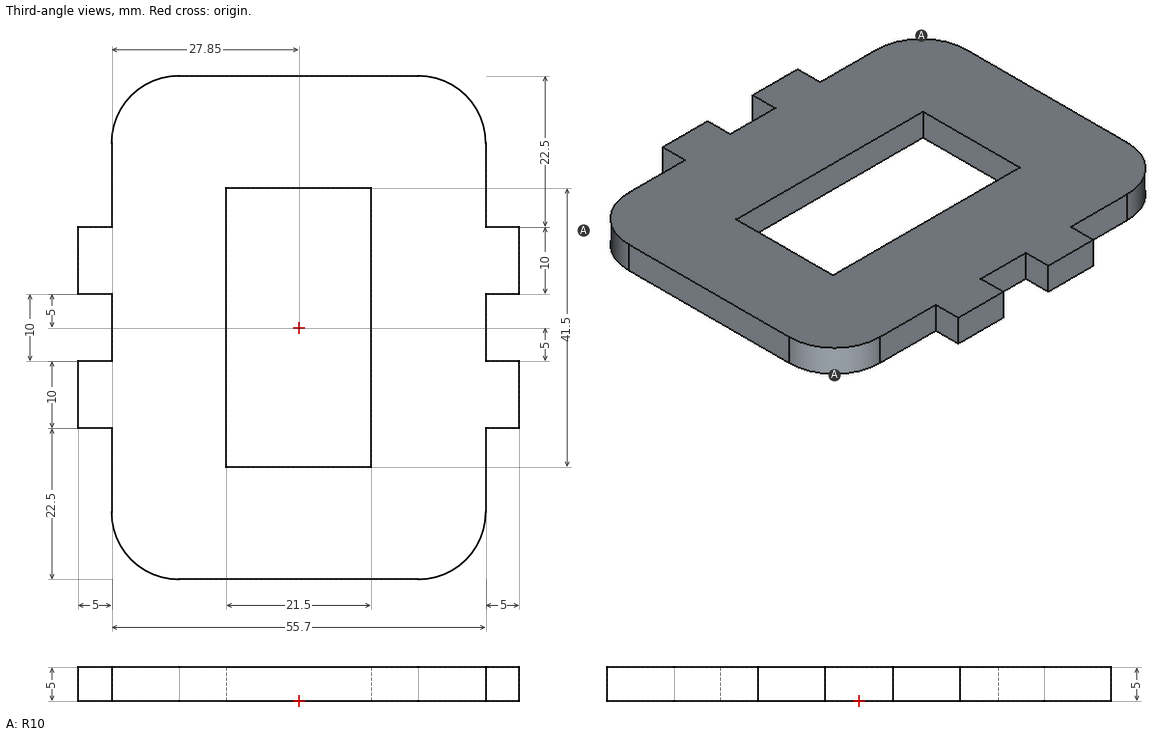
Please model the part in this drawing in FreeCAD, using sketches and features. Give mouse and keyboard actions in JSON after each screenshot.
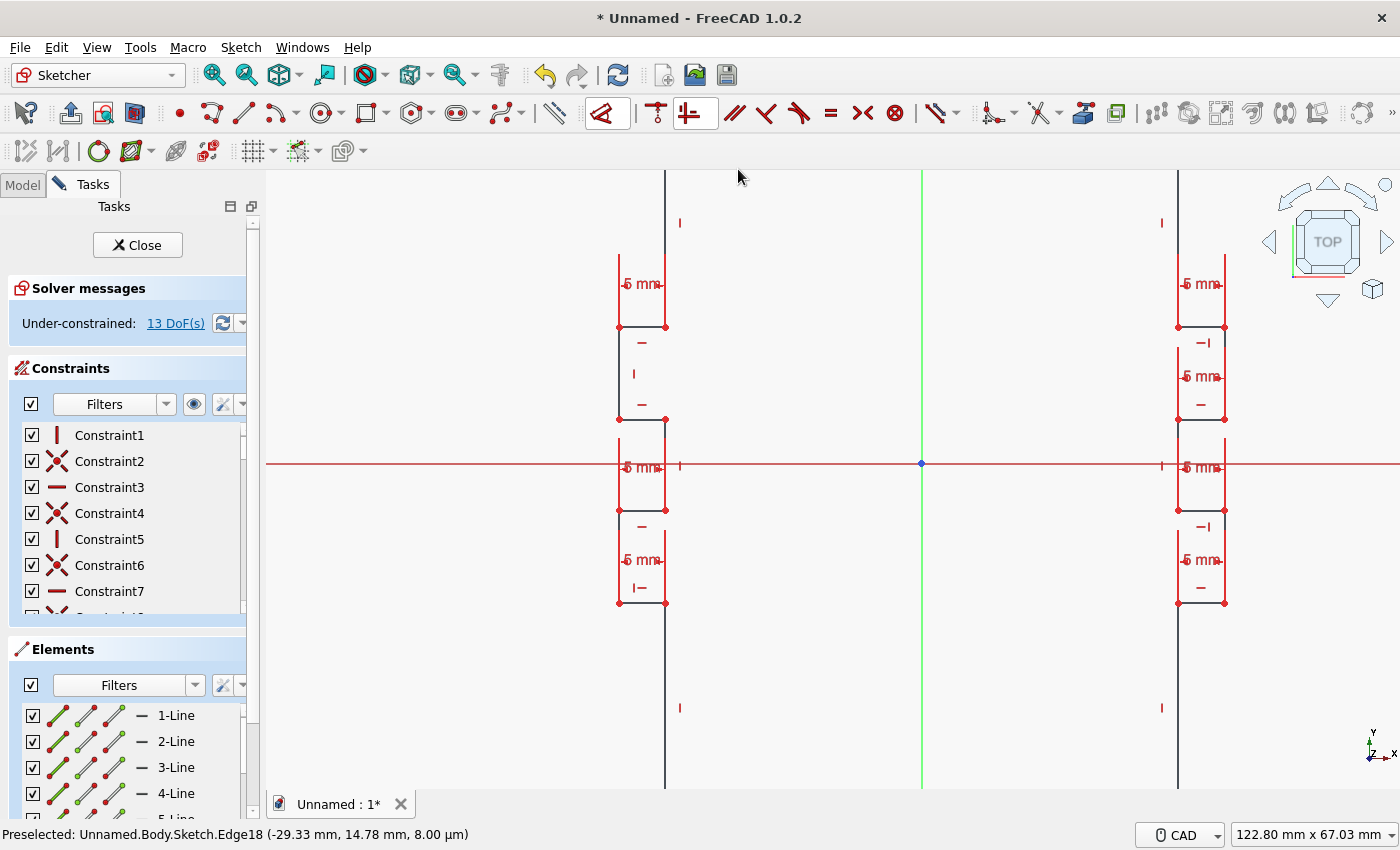
{"action": "left_click", "coordinate": [633, 420]}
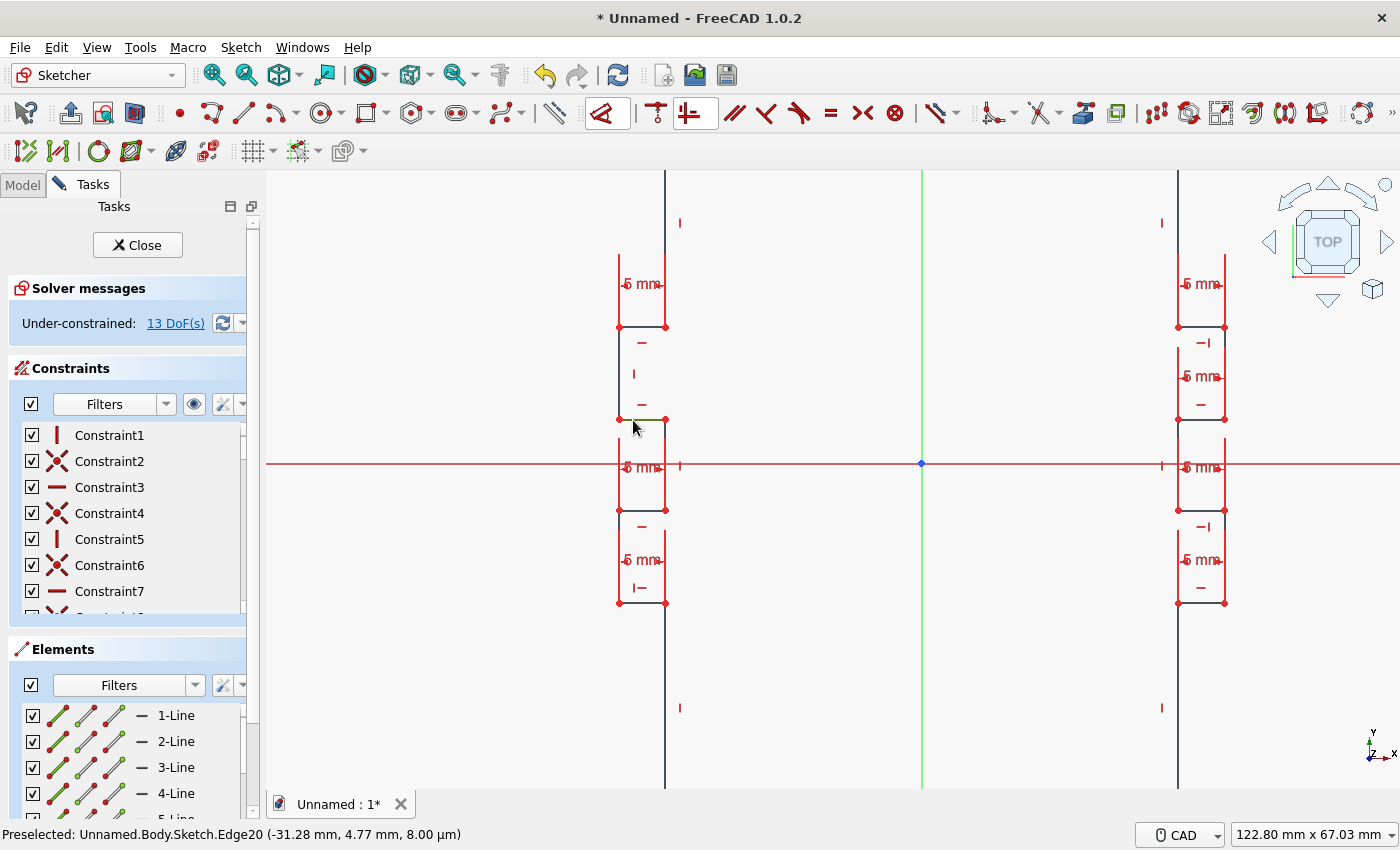
{"action": "key", "text": "l"}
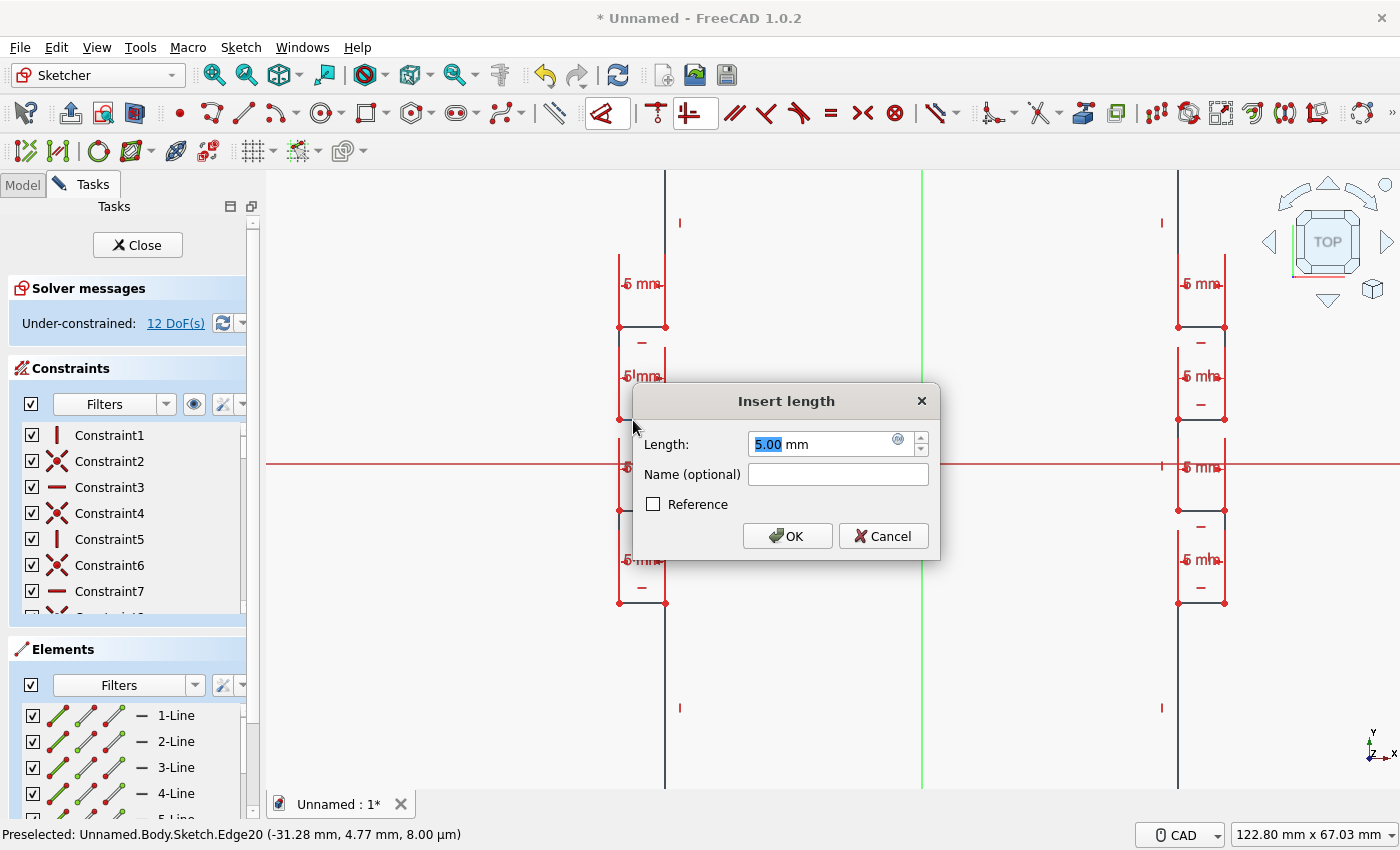
{"action": "type", "text": "5"}
{"action": "key", "text": "Return"}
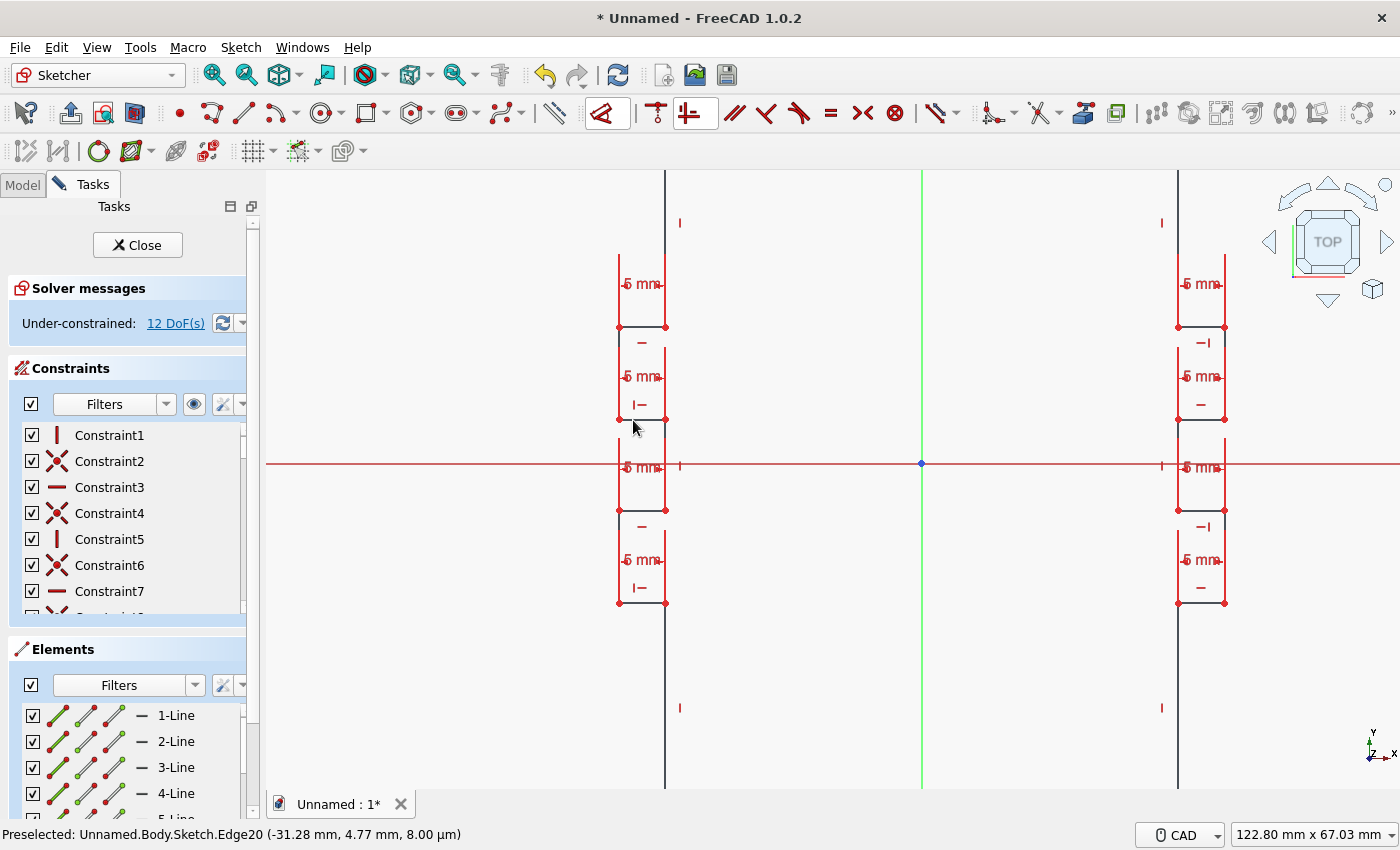
{"action": "left_click", "coordinate": [665, 447]}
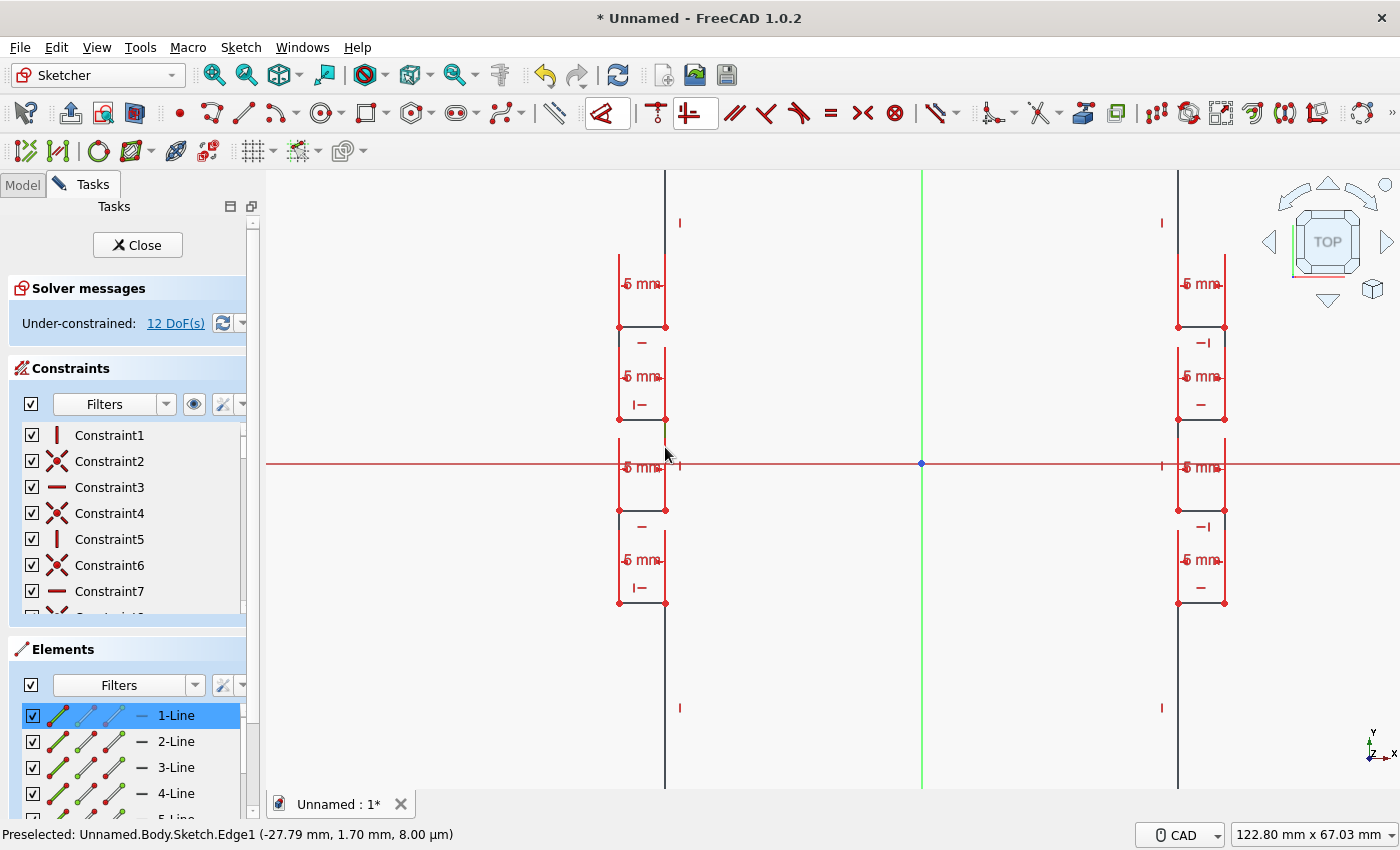
{"action": "left_click", "coordinate": [624, 114]}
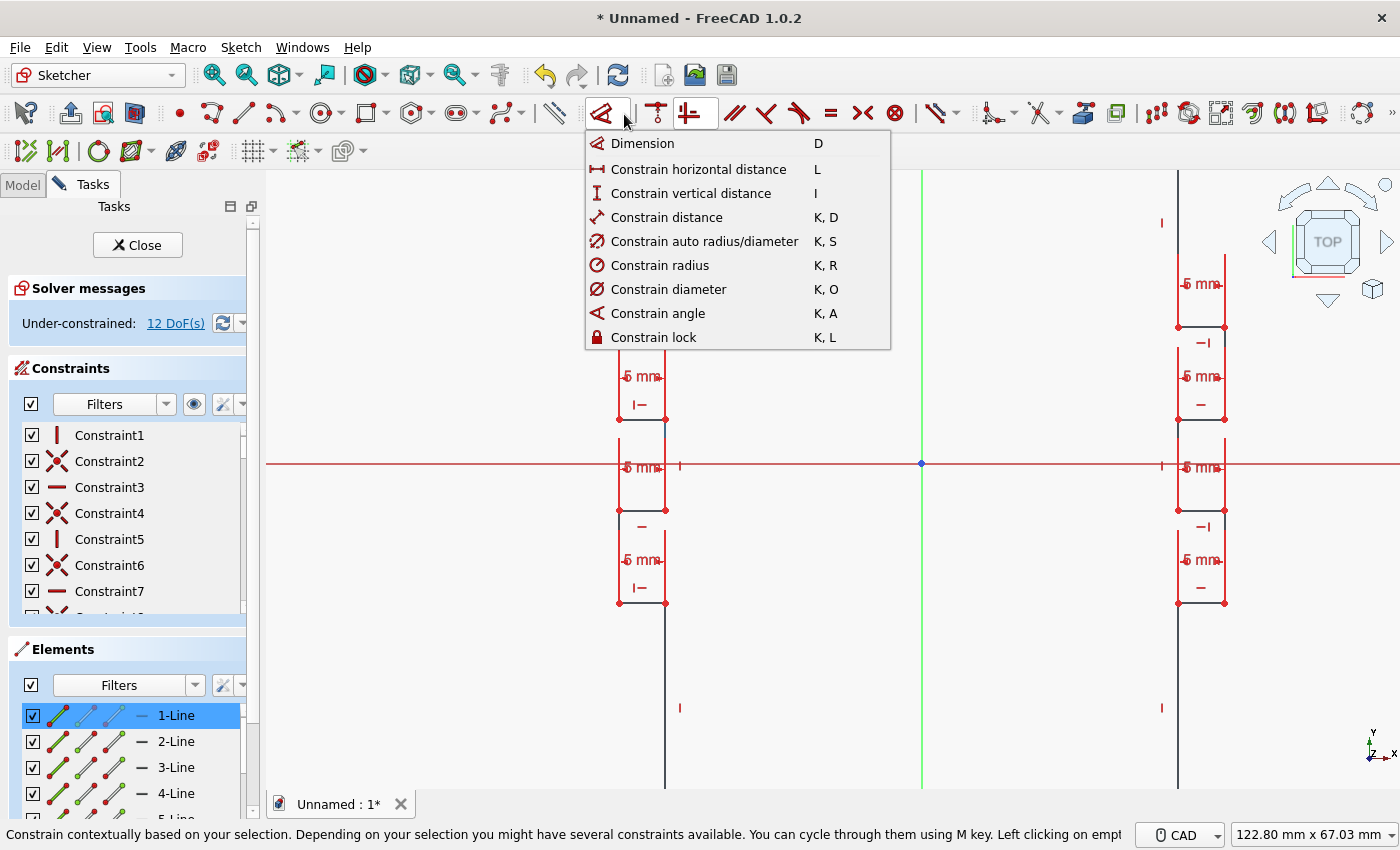
{"action": "left_click", "coordinate": [738, 193]}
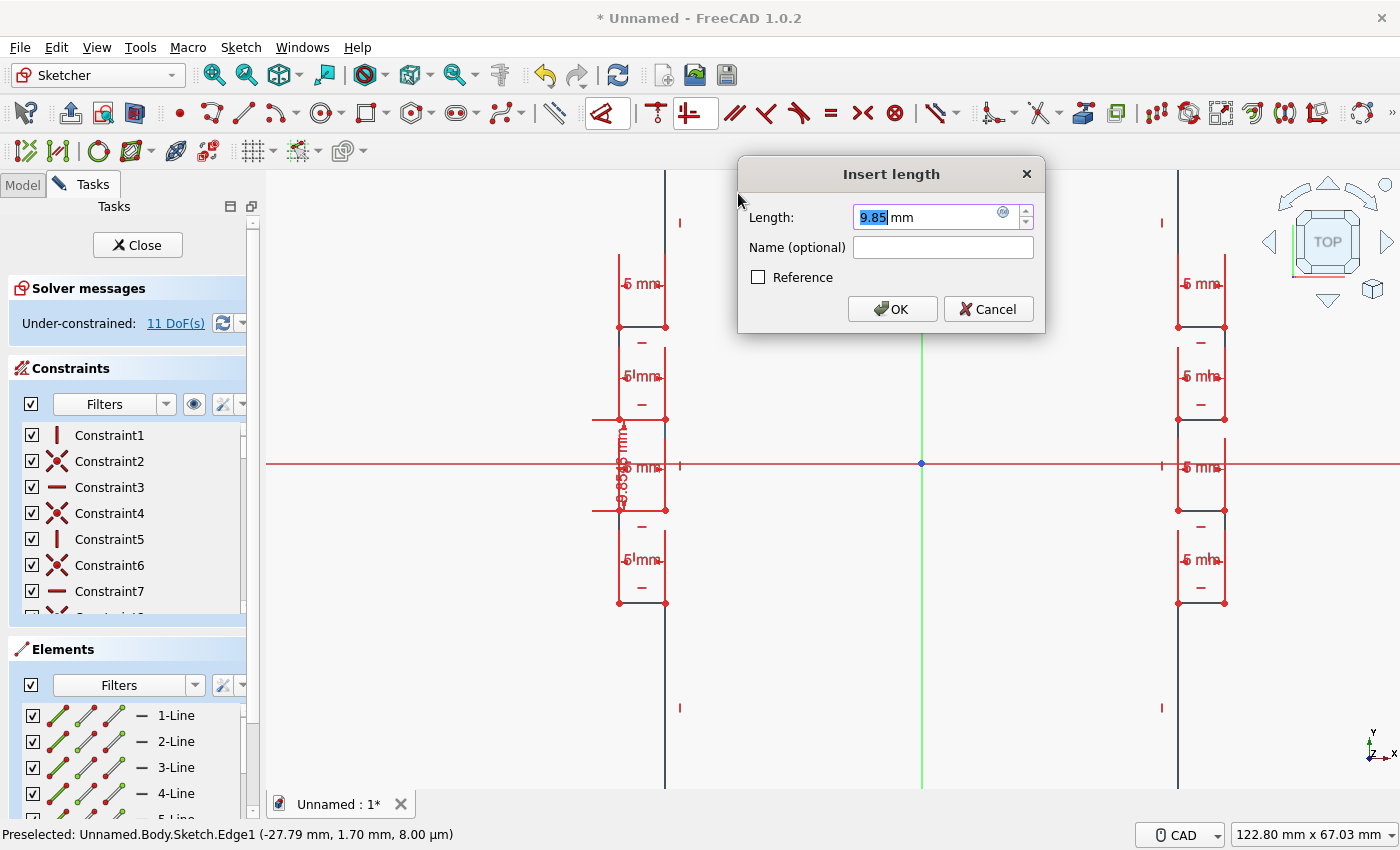
{"action": "type", "text": "10"}
{"action": "key", "text": "Return"}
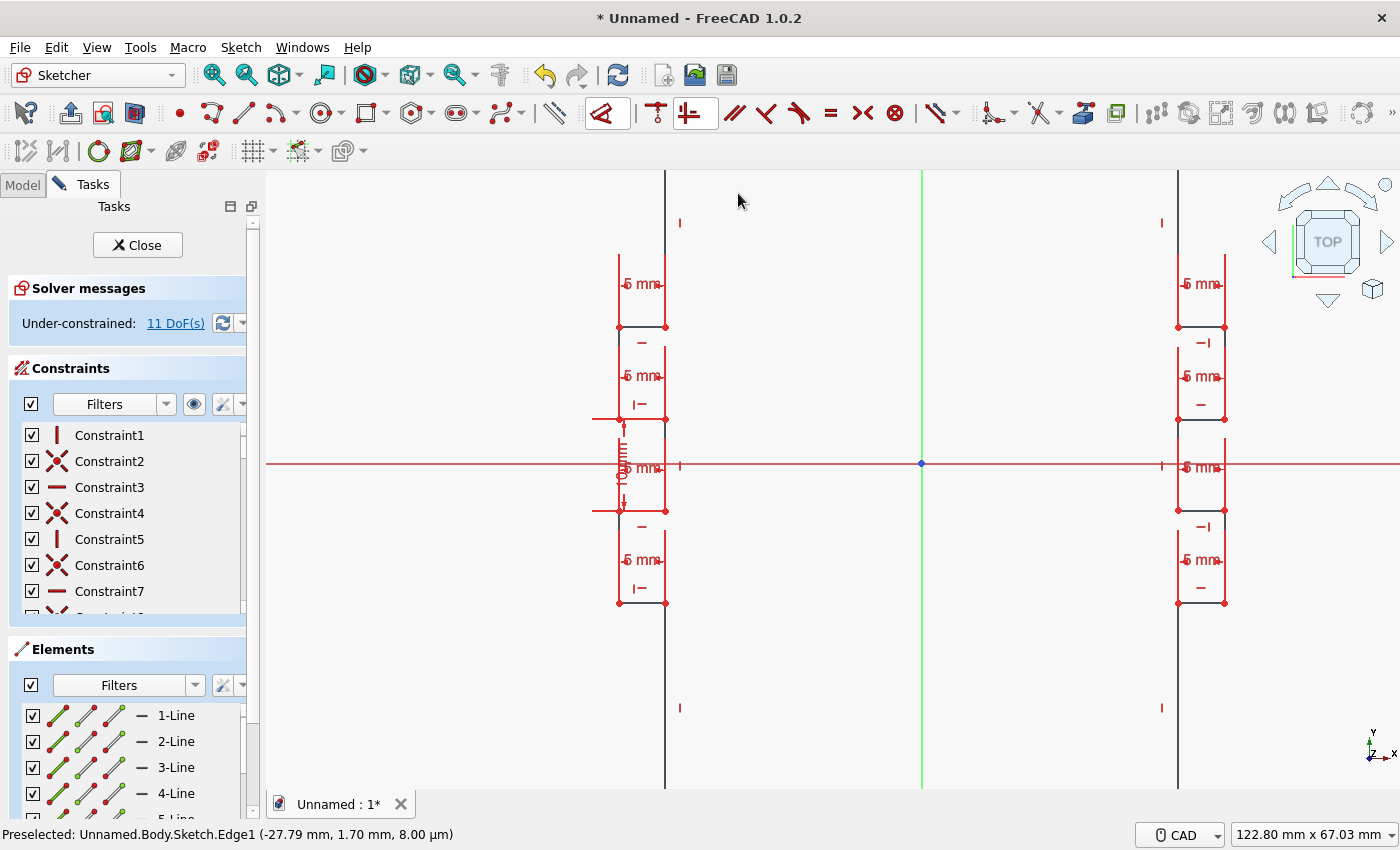
{"action": "left_click", "coordinate": [619, 539]}